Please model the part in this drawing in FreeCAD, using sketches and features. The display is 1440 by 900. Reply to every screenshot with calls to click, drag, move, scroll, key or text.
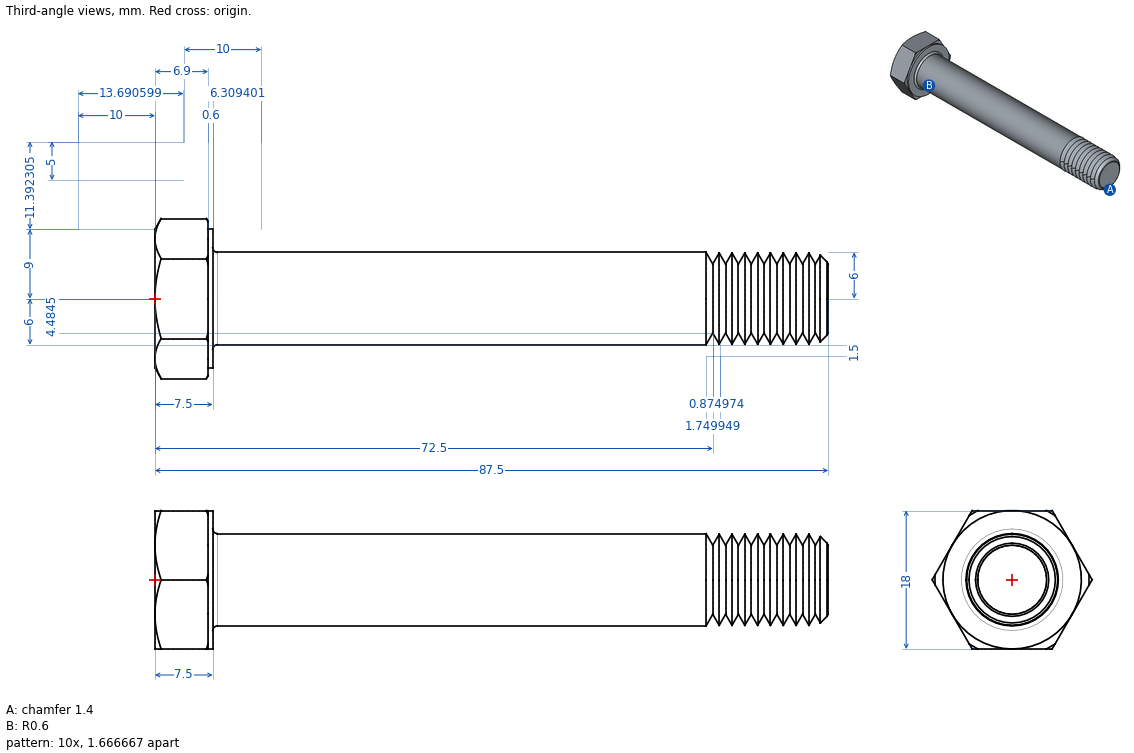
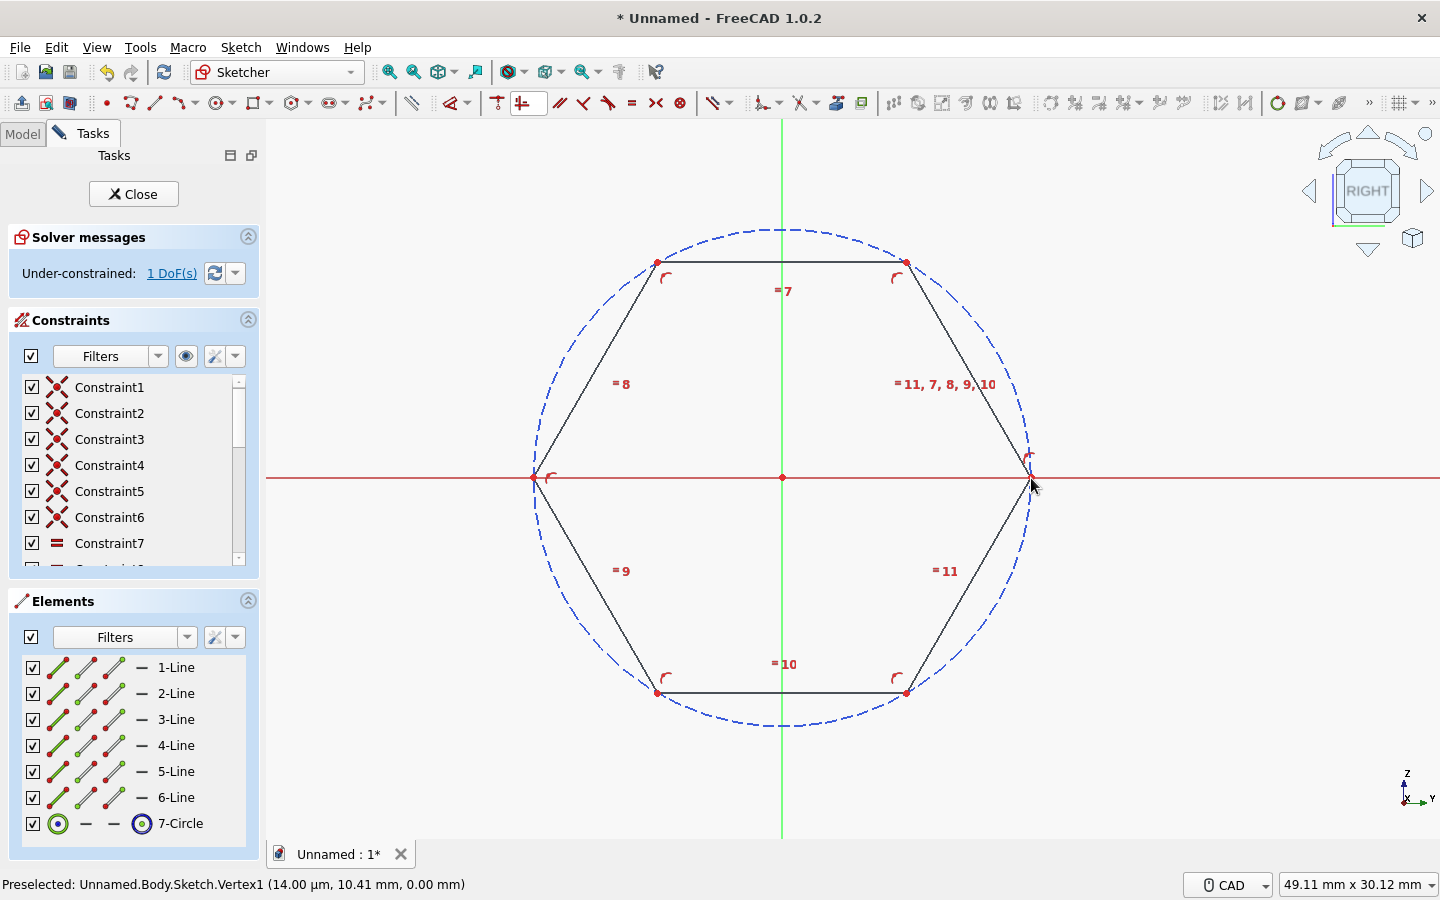
click(450, 104)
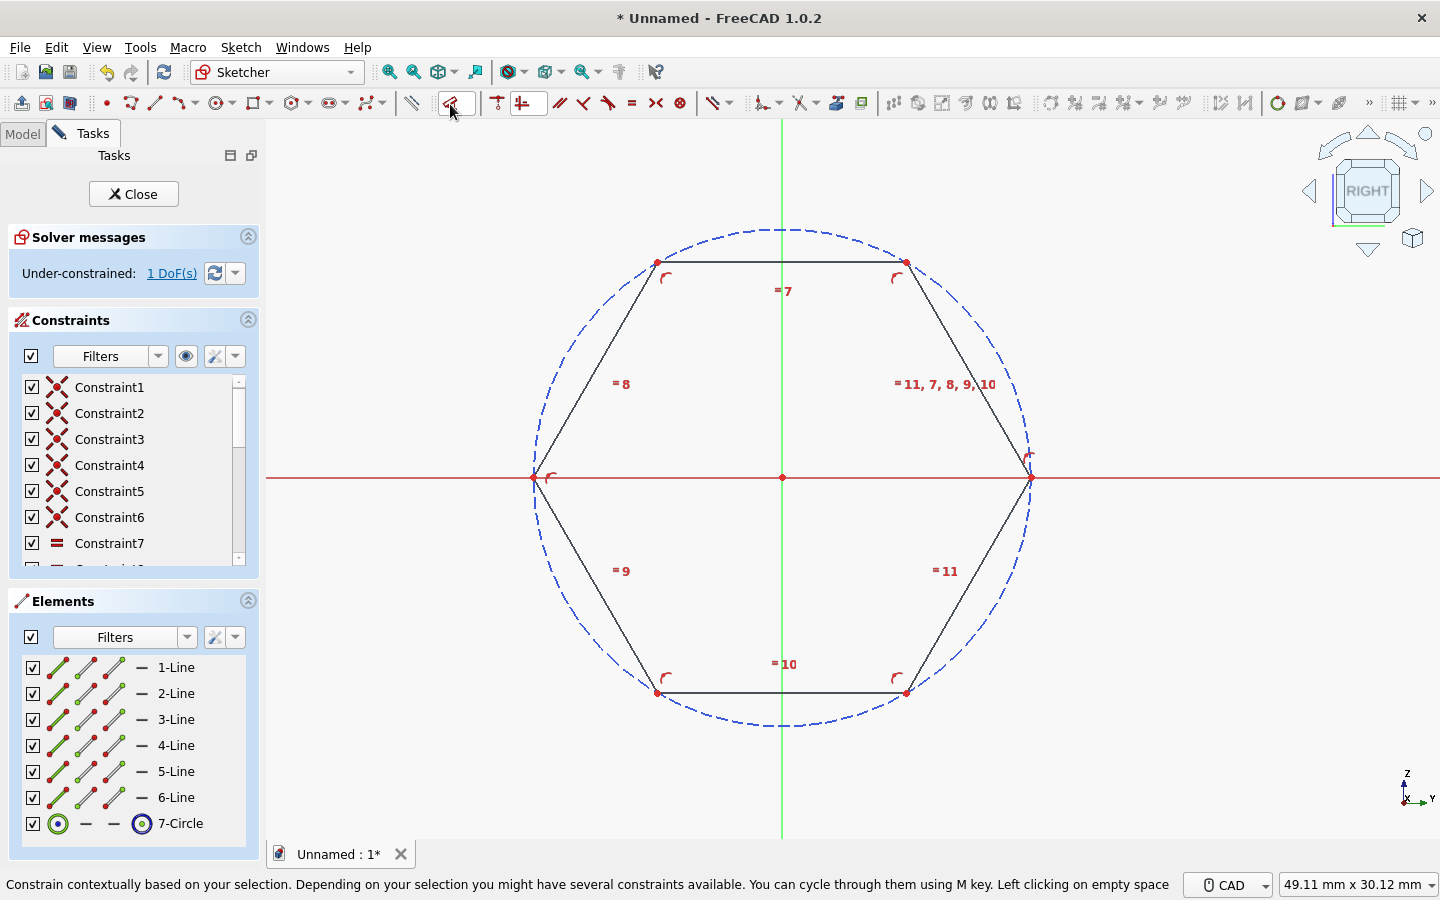
click(658, 693)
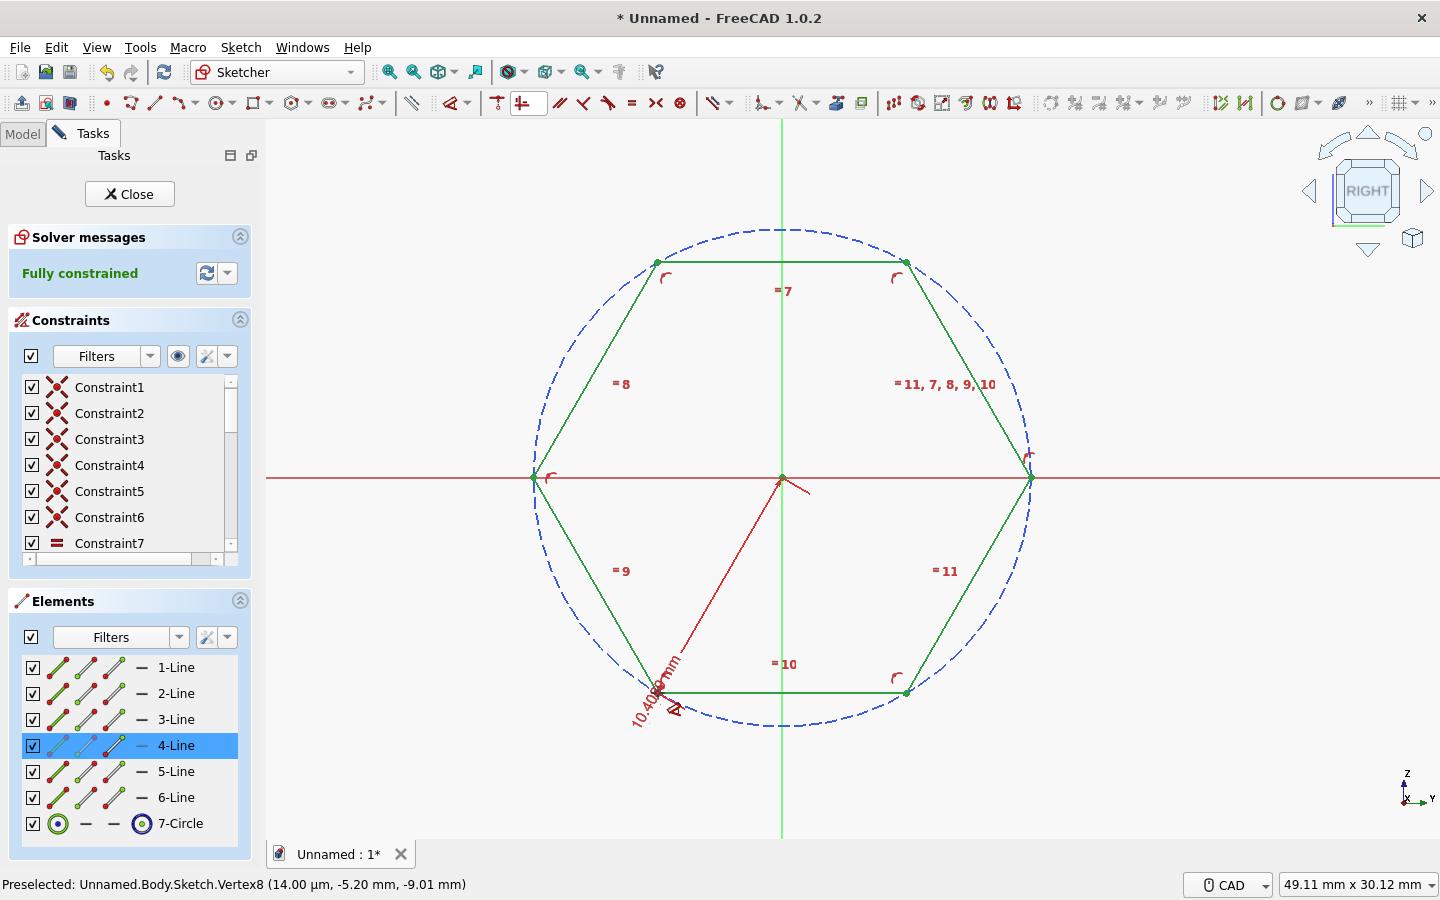
click(907, 262)
click(941, 379)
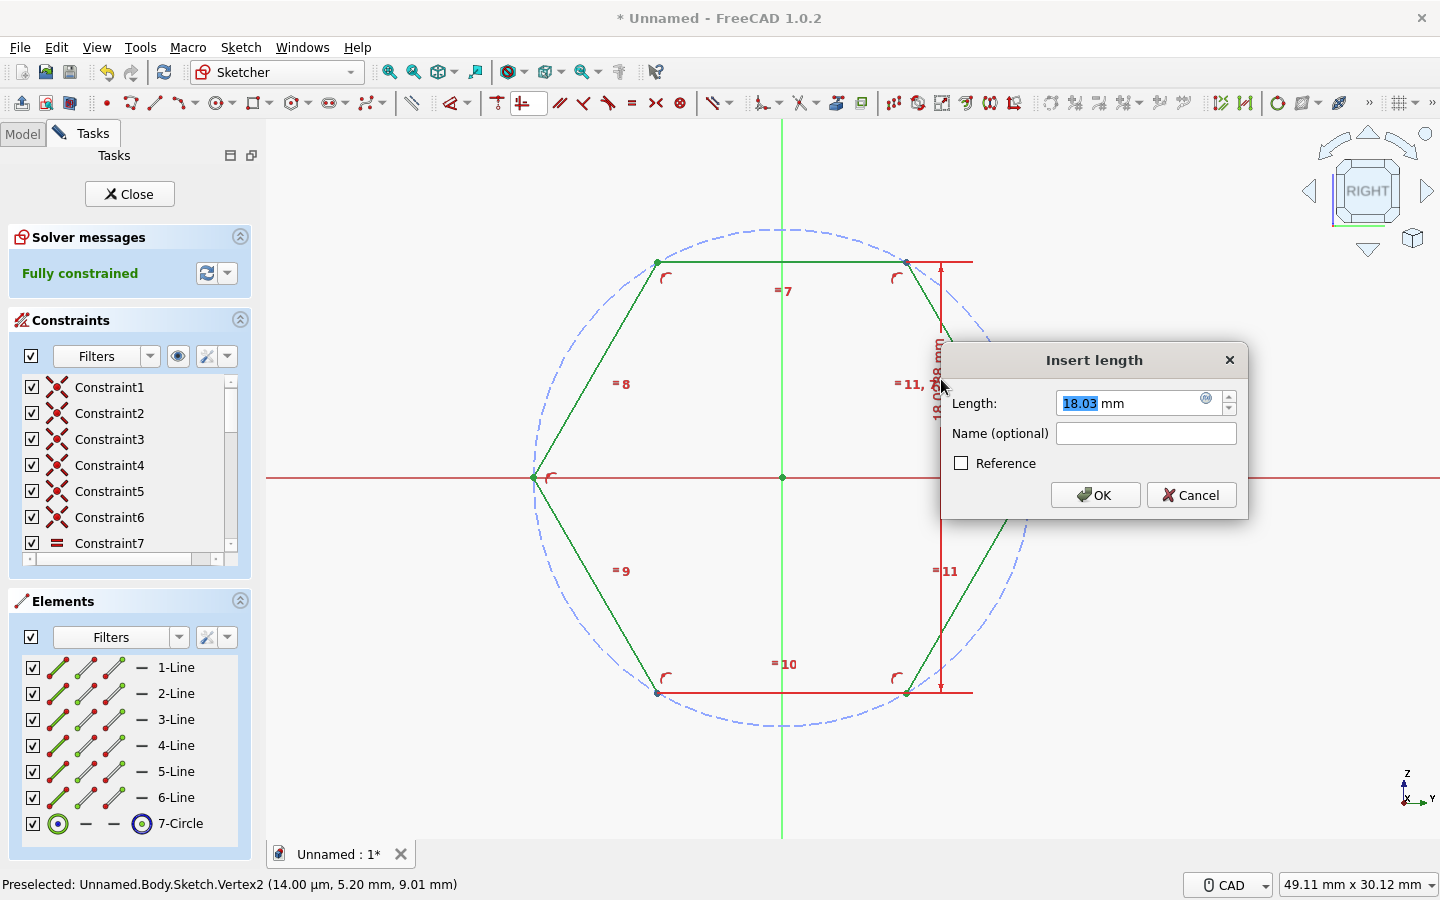
text(18)
key(Return)
key(Escape)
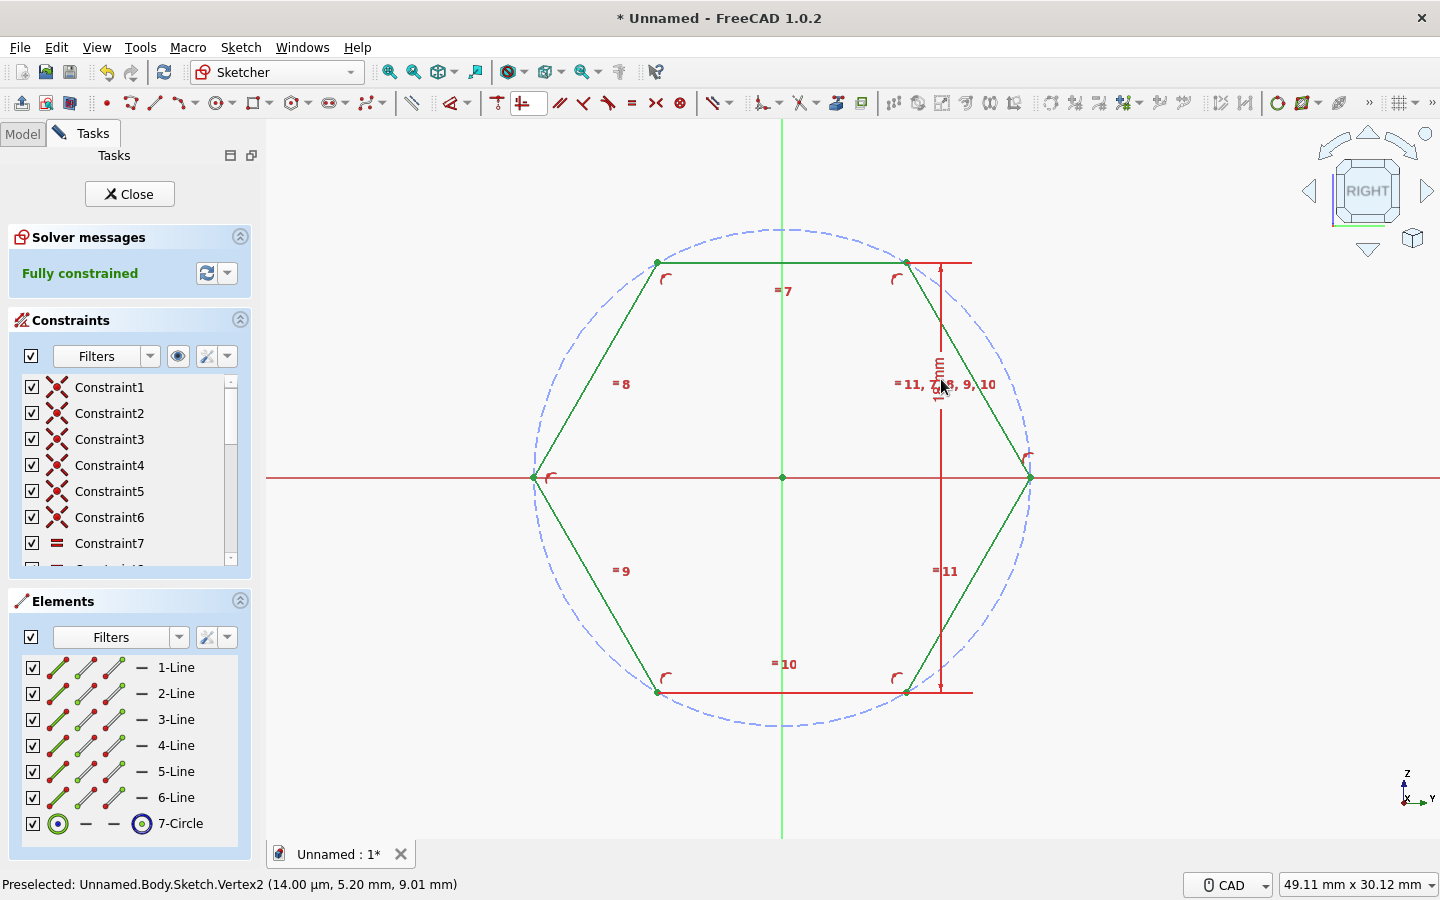
click(130, 194)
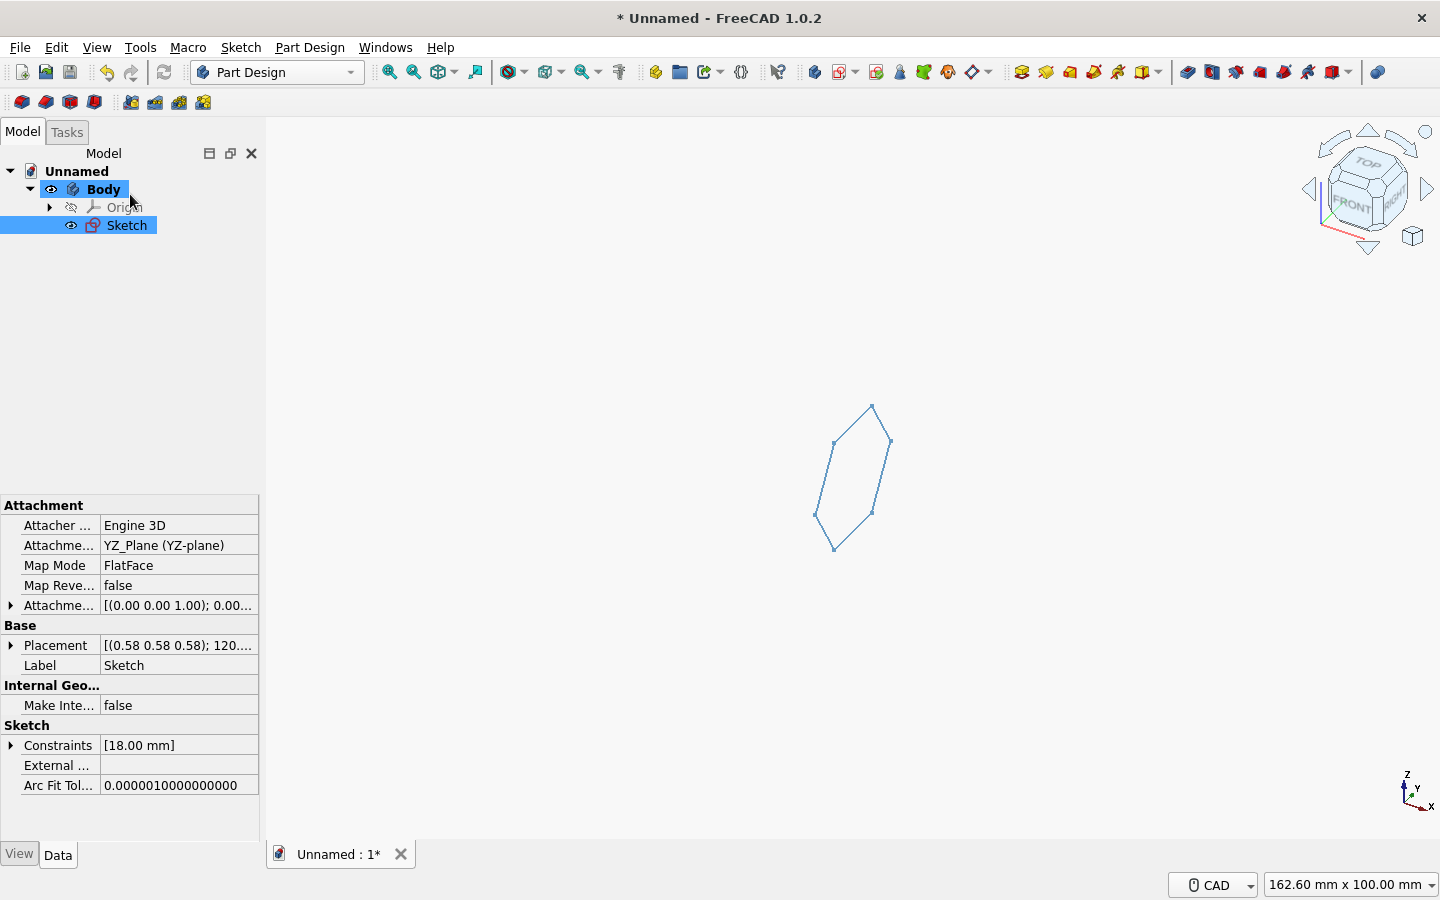
click(1022, 72)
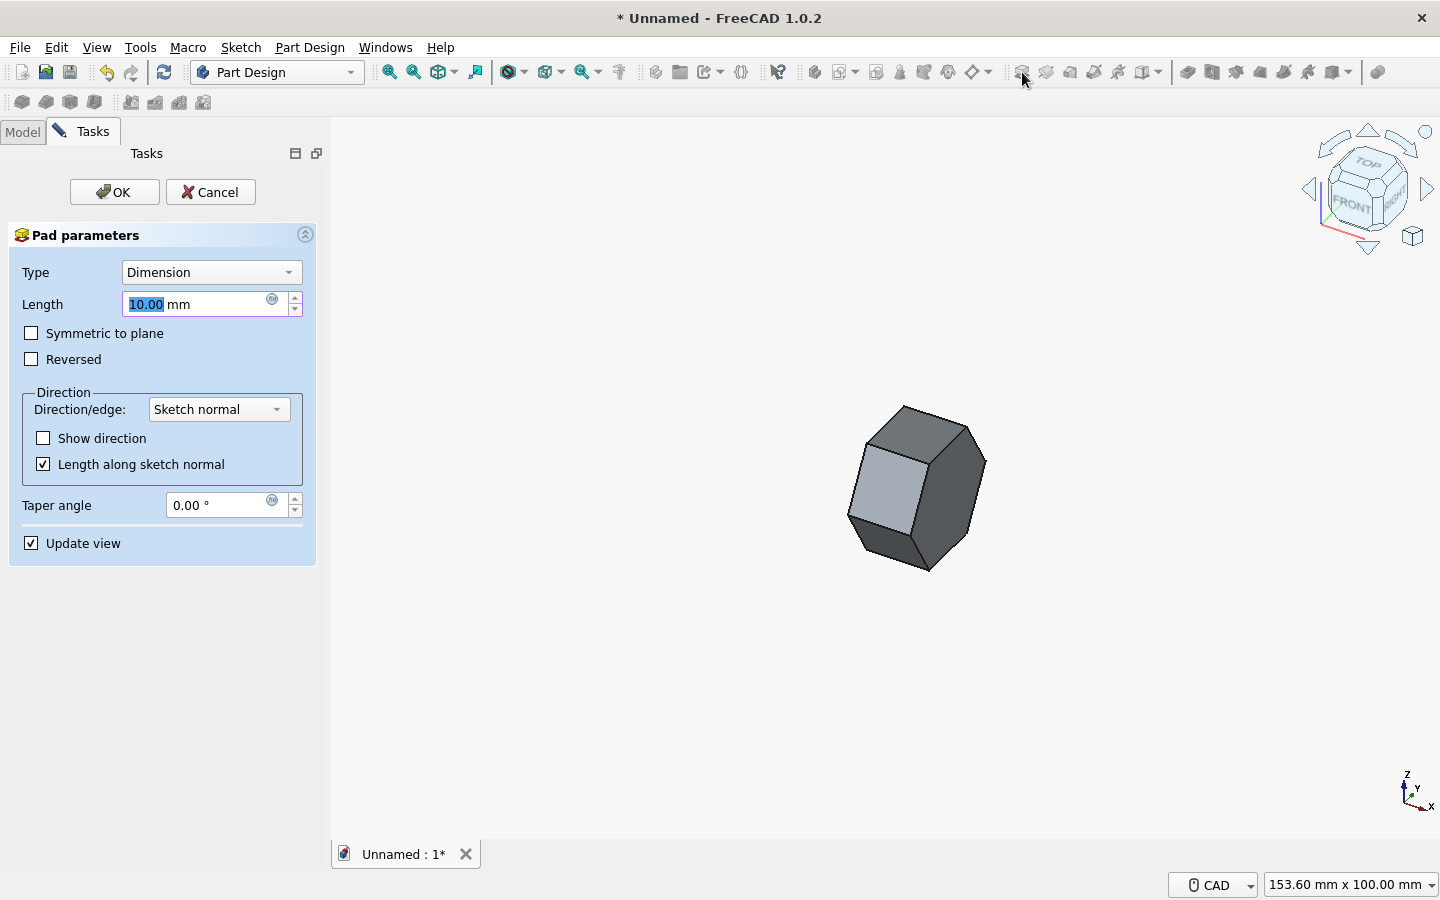
text(7.5)
key(Tab)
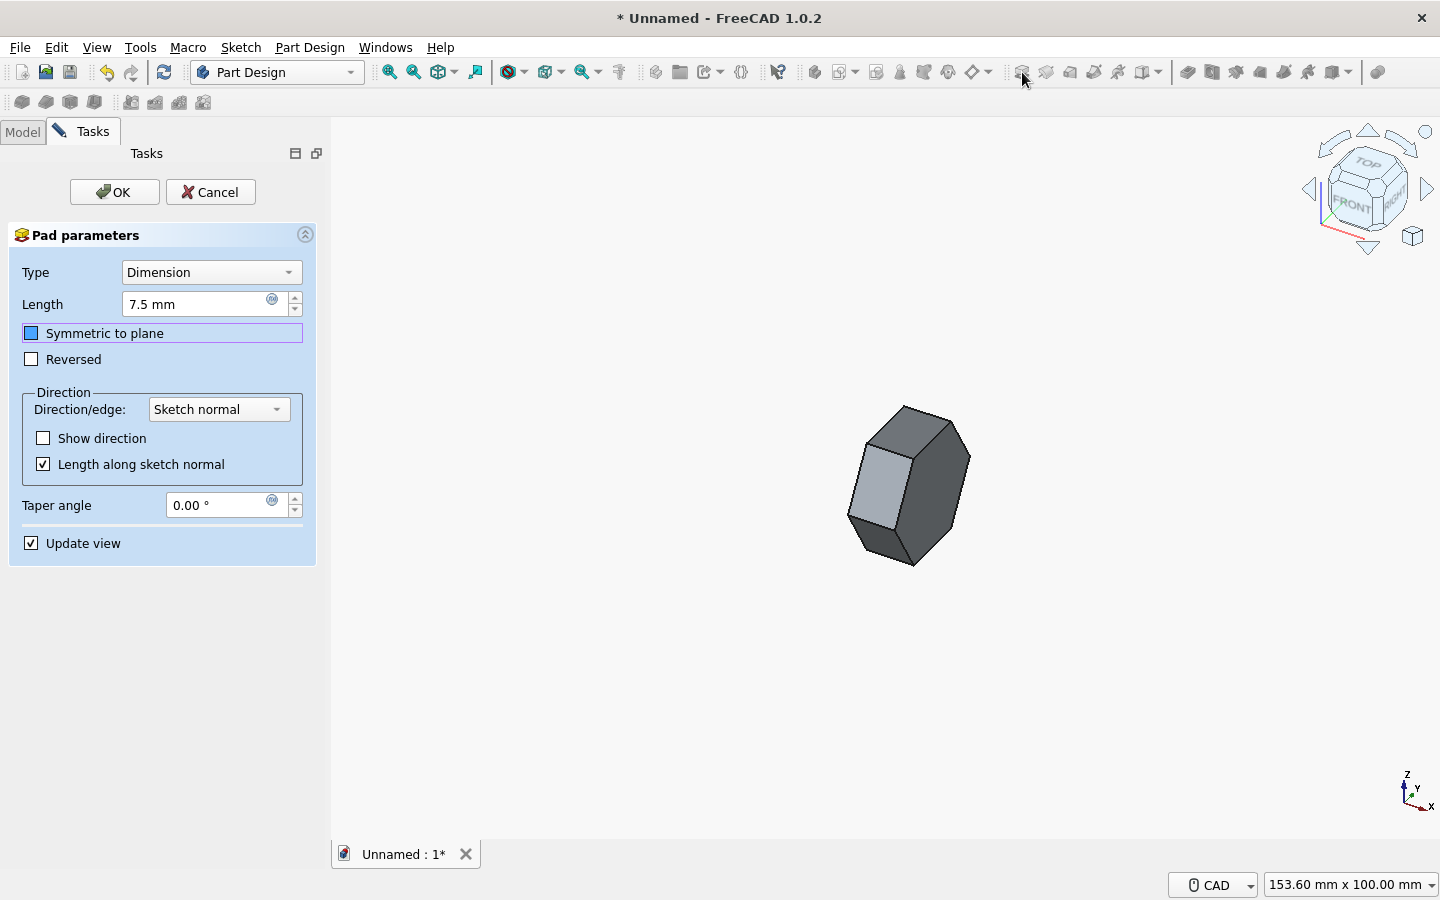
click(115, 192)